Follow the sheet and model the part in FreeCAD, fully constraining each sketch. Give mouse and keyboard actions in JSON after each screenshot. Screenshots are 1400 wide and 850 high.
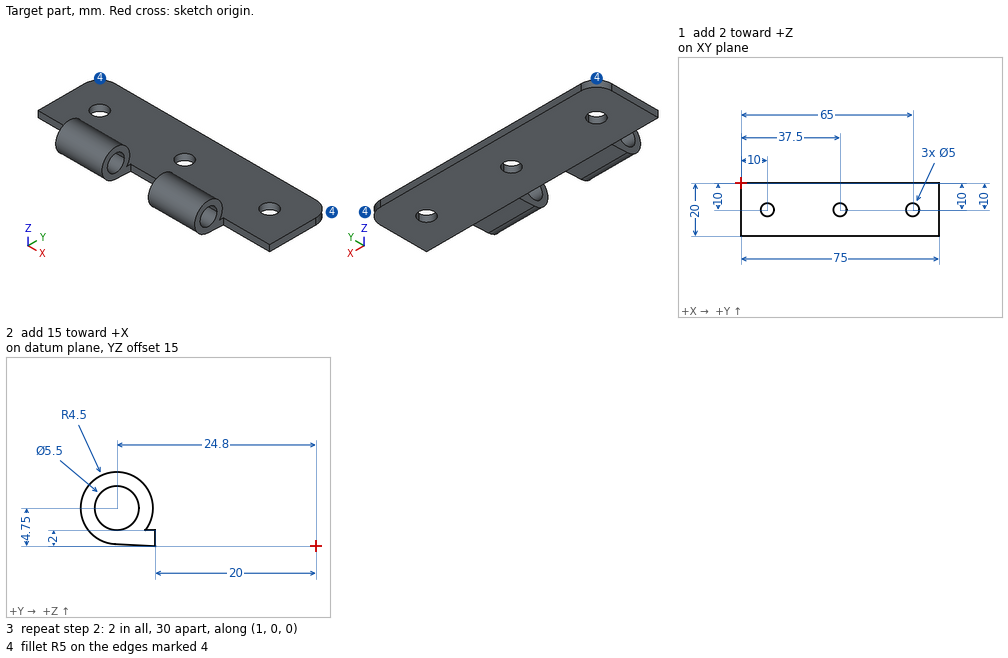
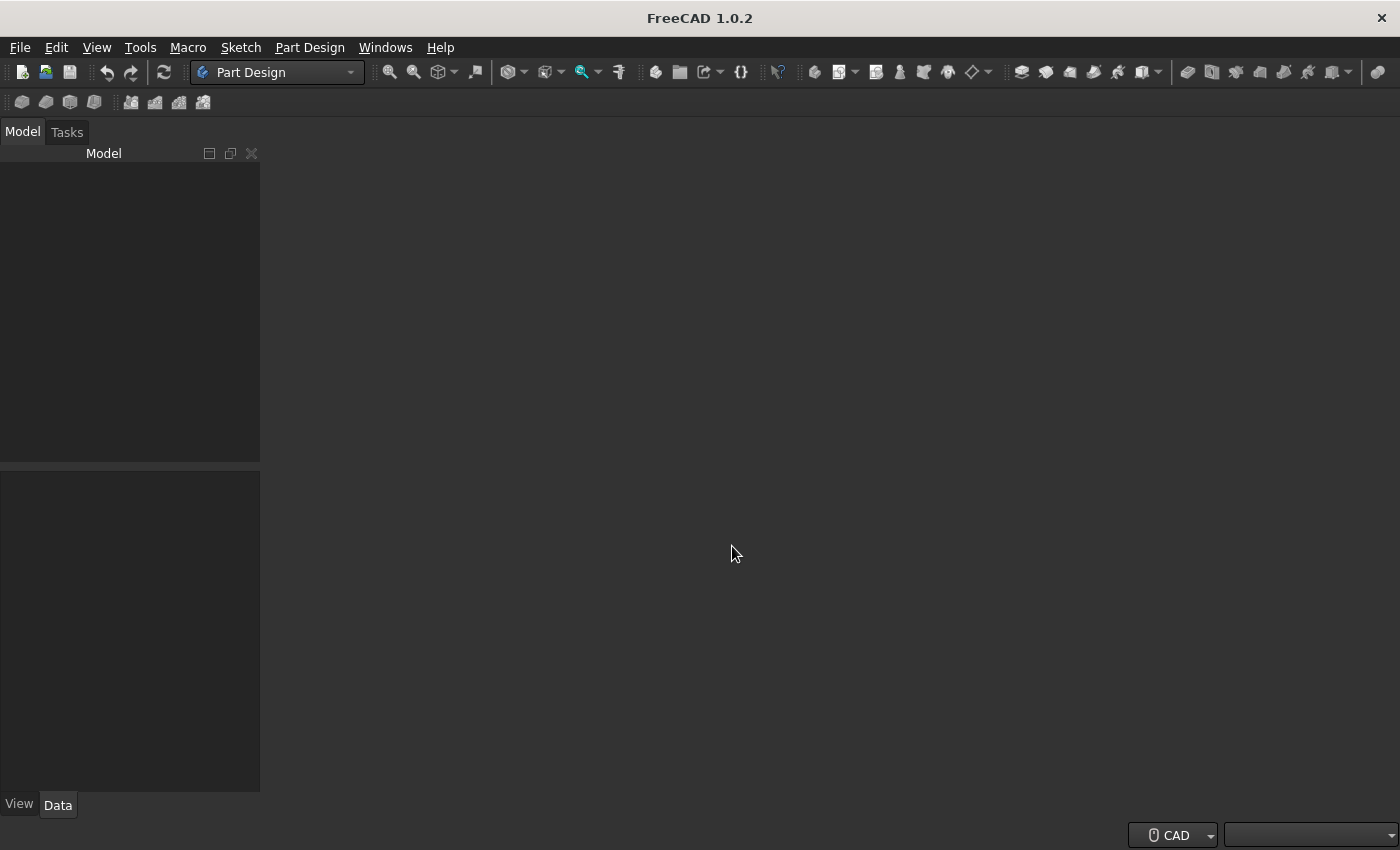
{"action": "left_click", "coordinate": [22, 72]}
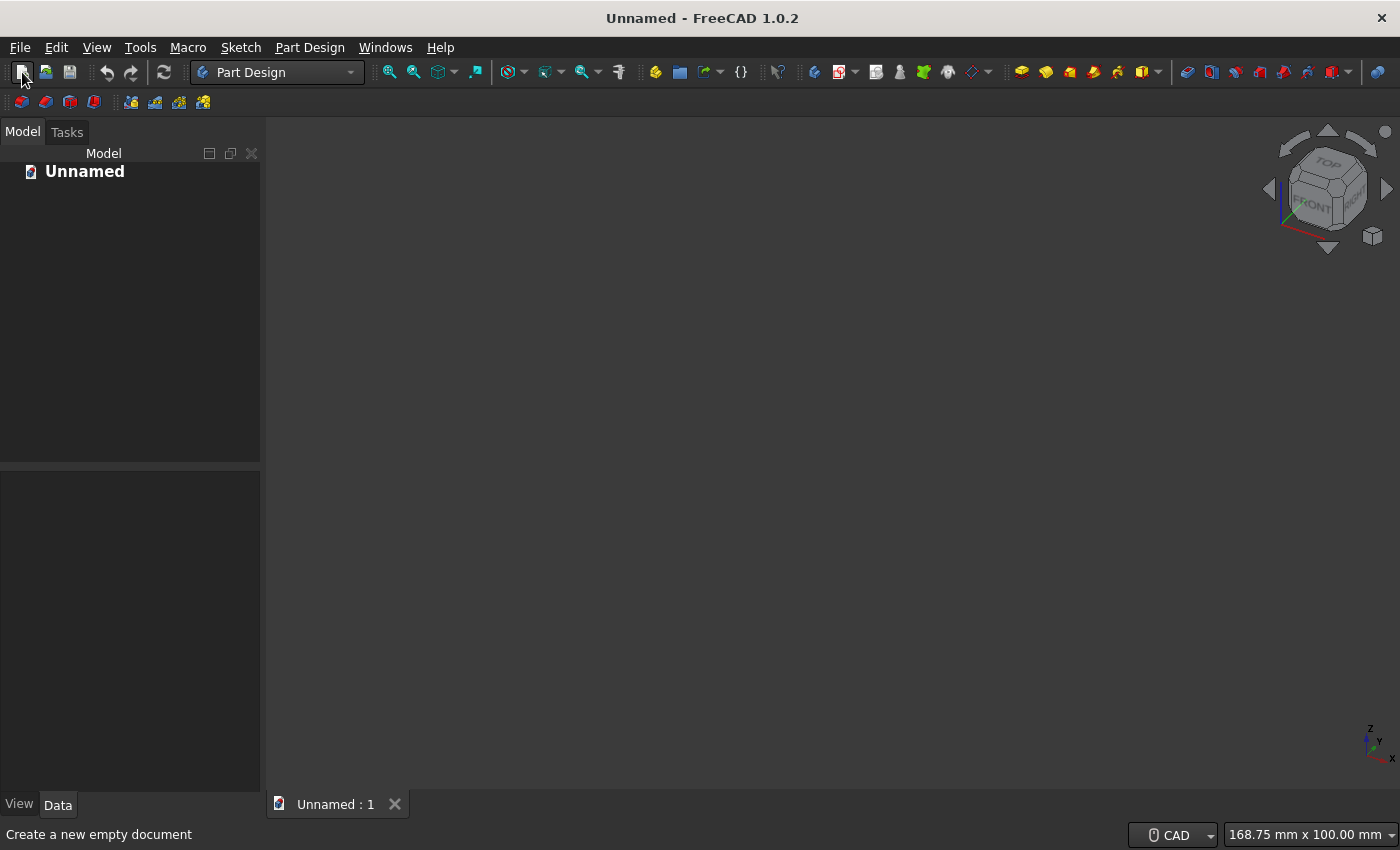
{"action": "left_click", "coordinate": [840, 72]}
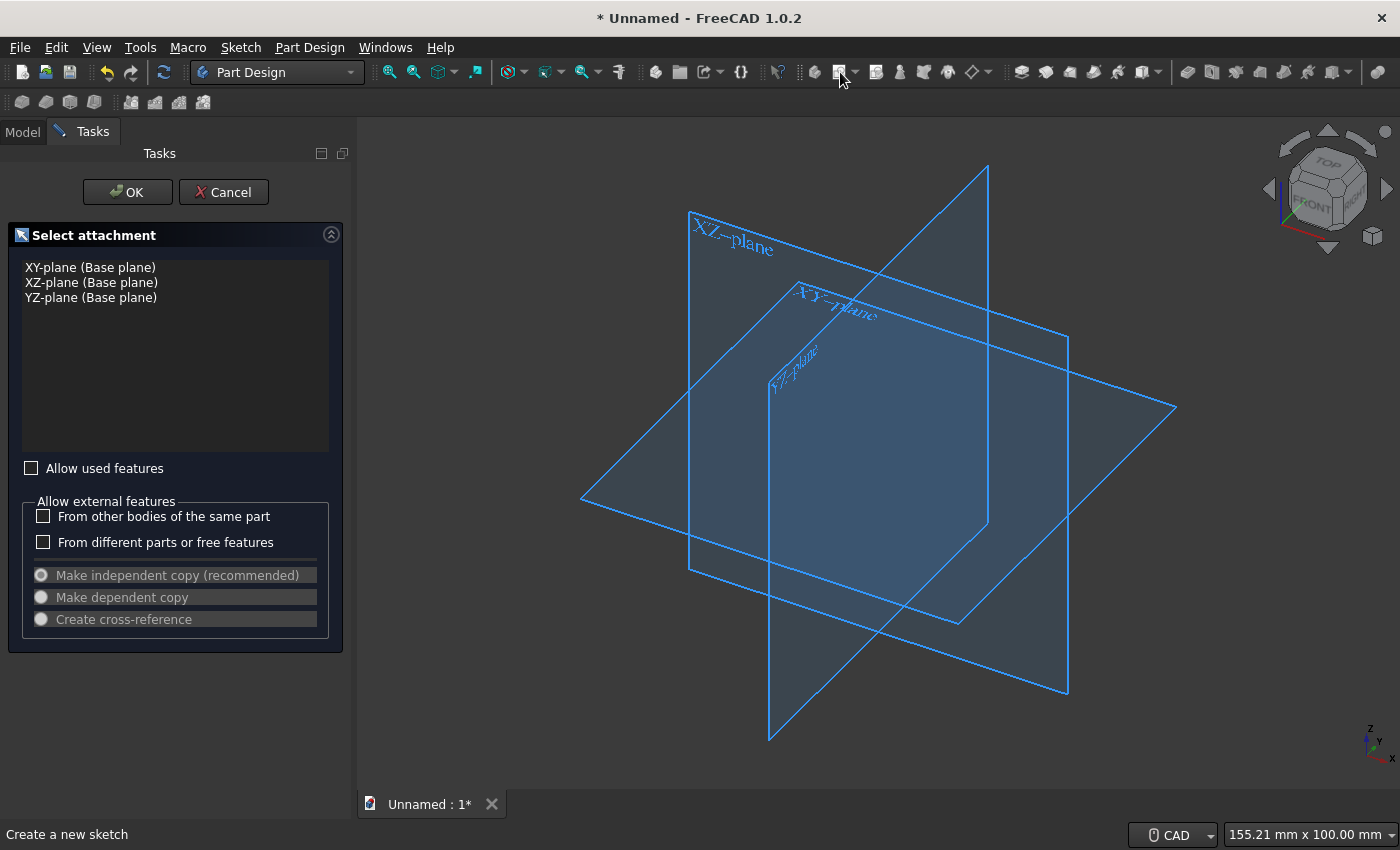
{"action": "left_click", "coordinate": [82, 268]}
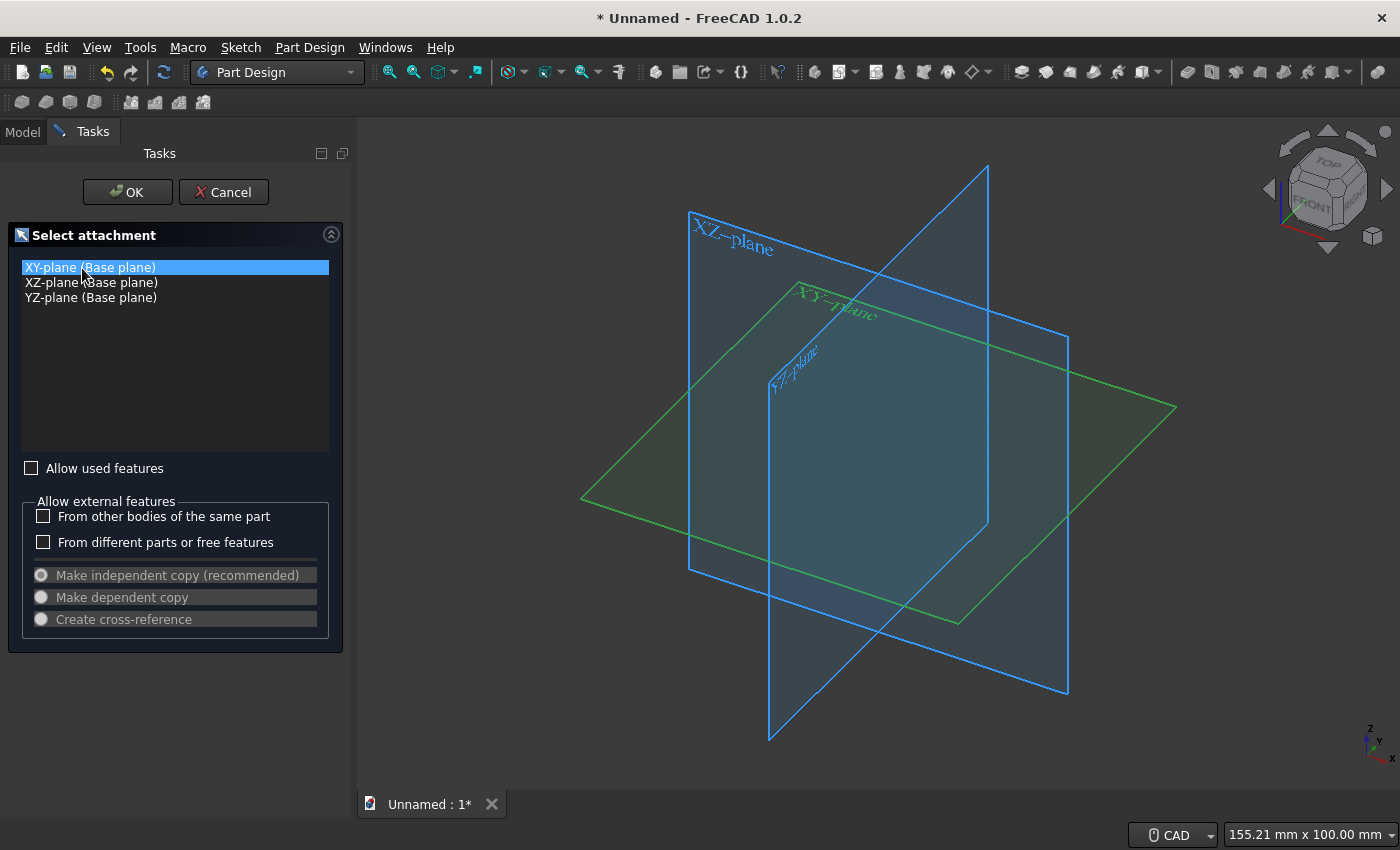
{"action": "left_click", "coordinate": [128, 192]}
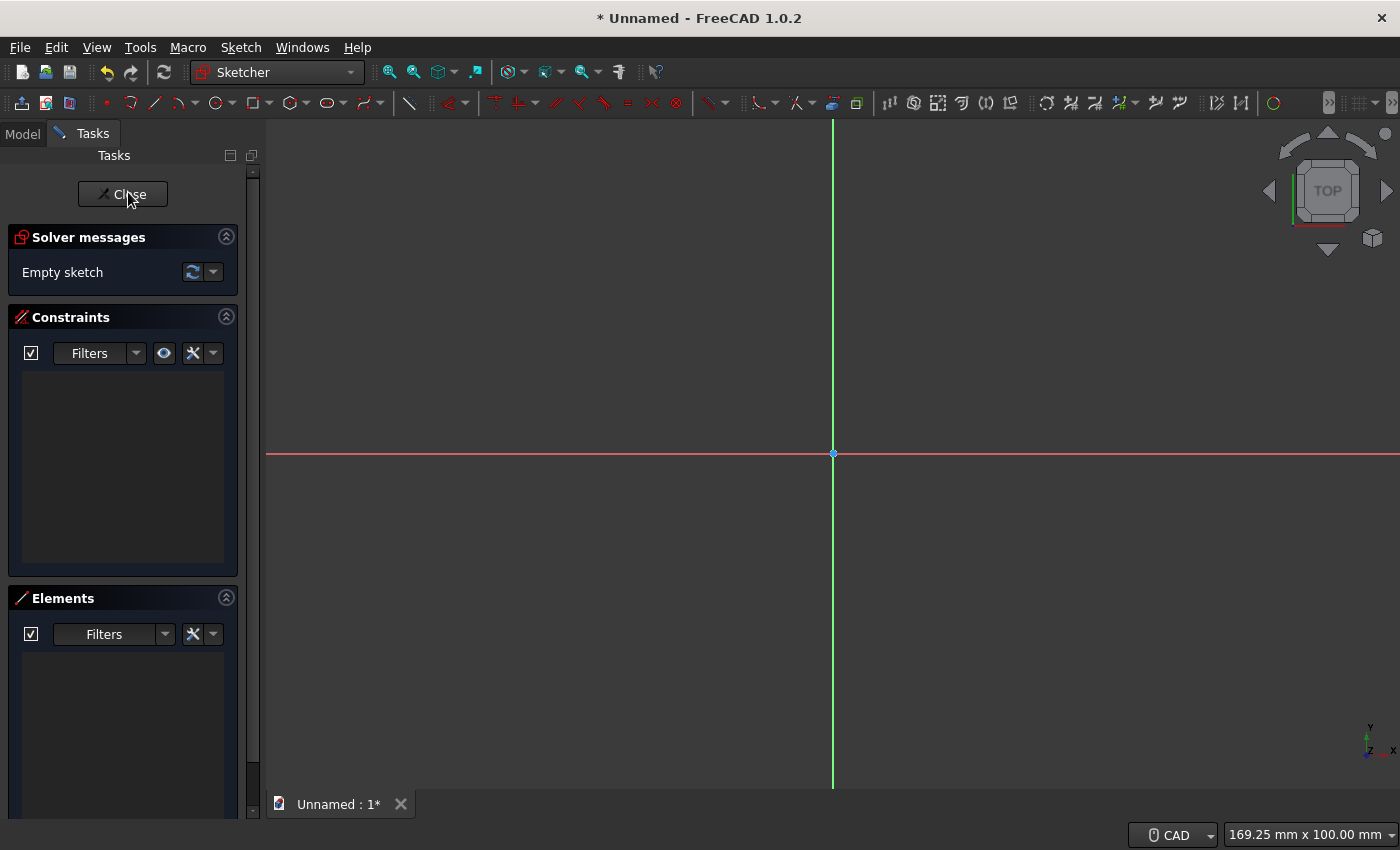
{"action": "scroll", "coordinate": [294, 151], "scroll_direction": "down", "scroll_amount": 1}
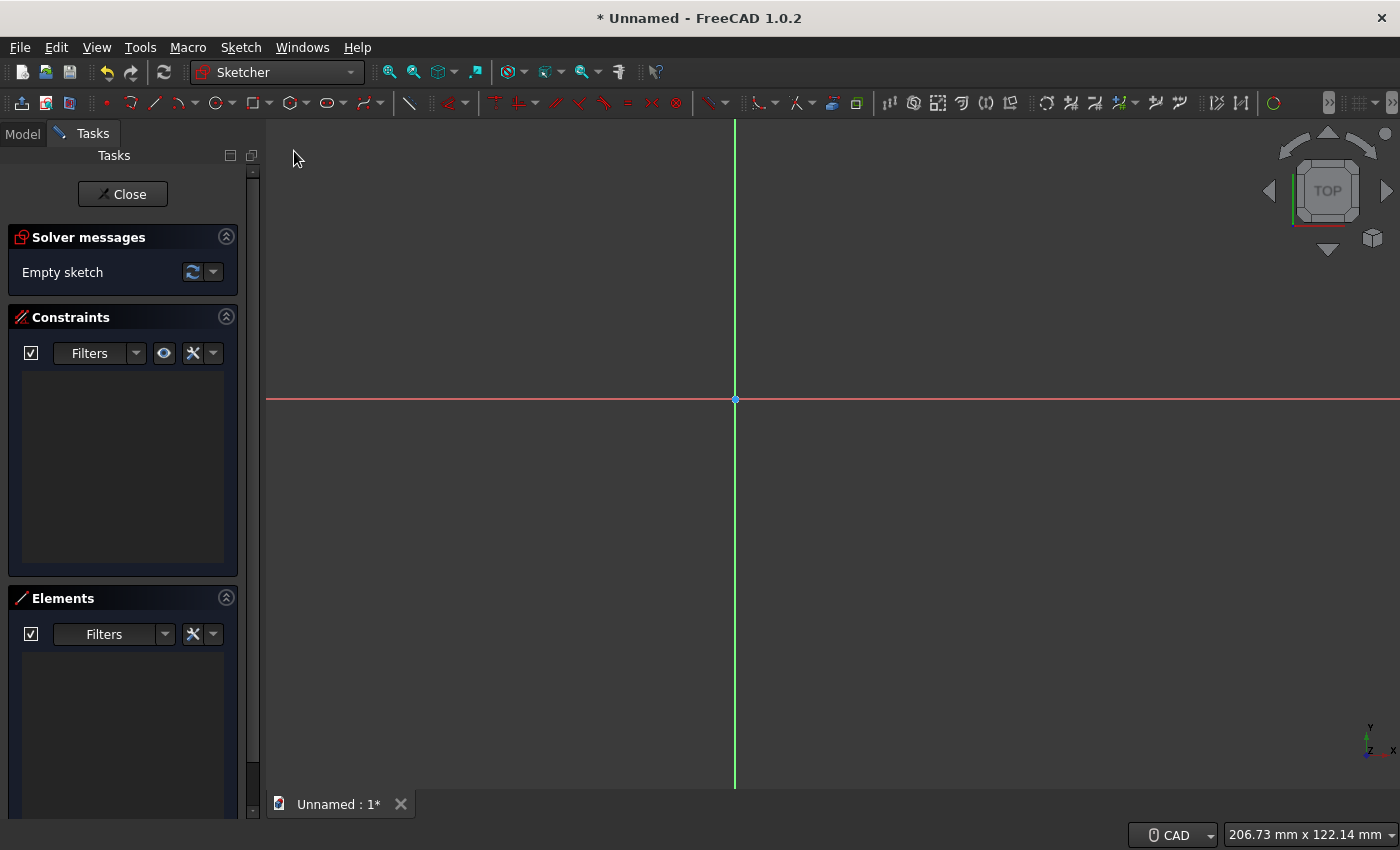
{"action": "scroll", "coordinate": [1235, 454], "scroll_direction": "up", "scroll_amount": 2}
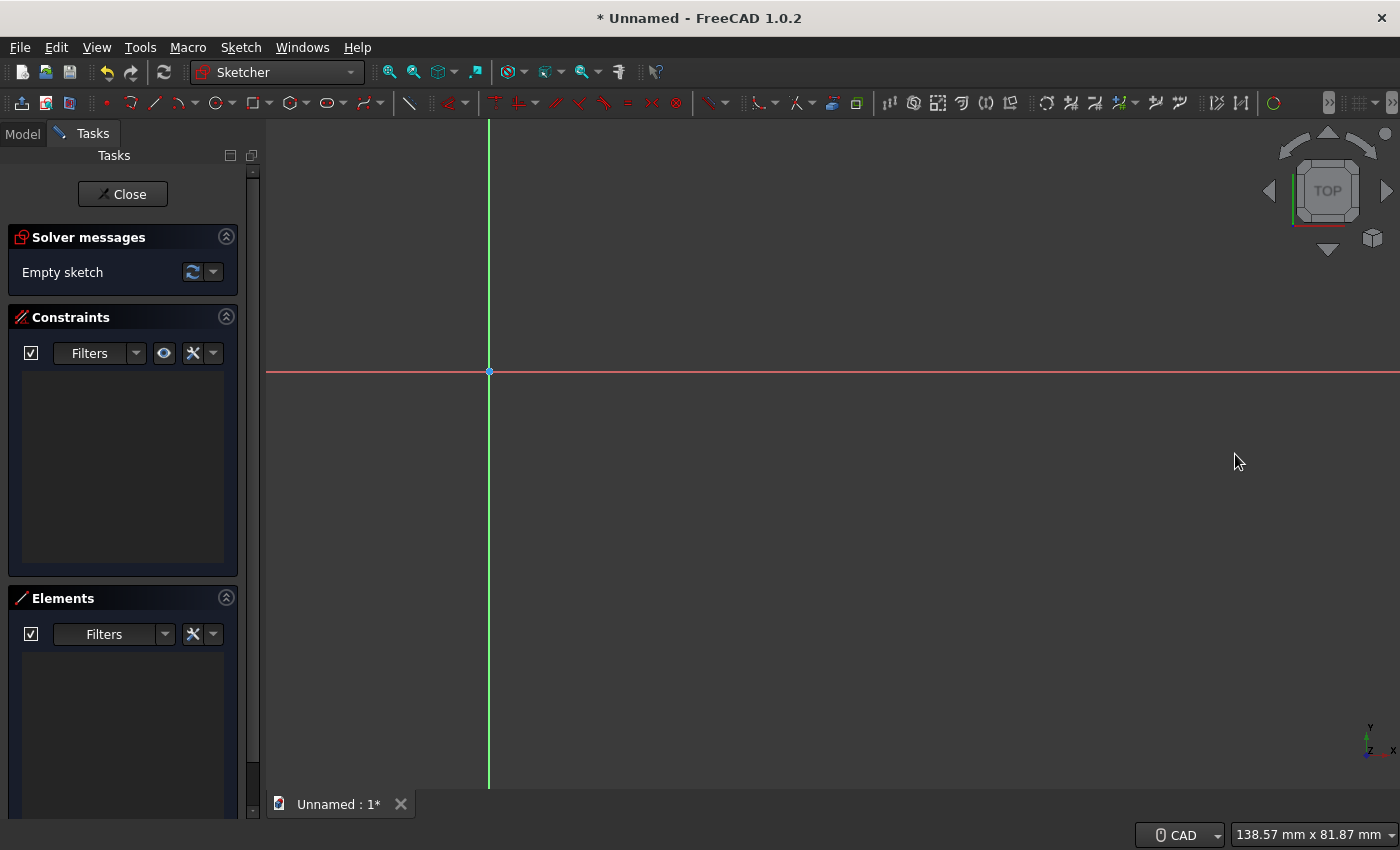
{"action": "key", "text": "g r"}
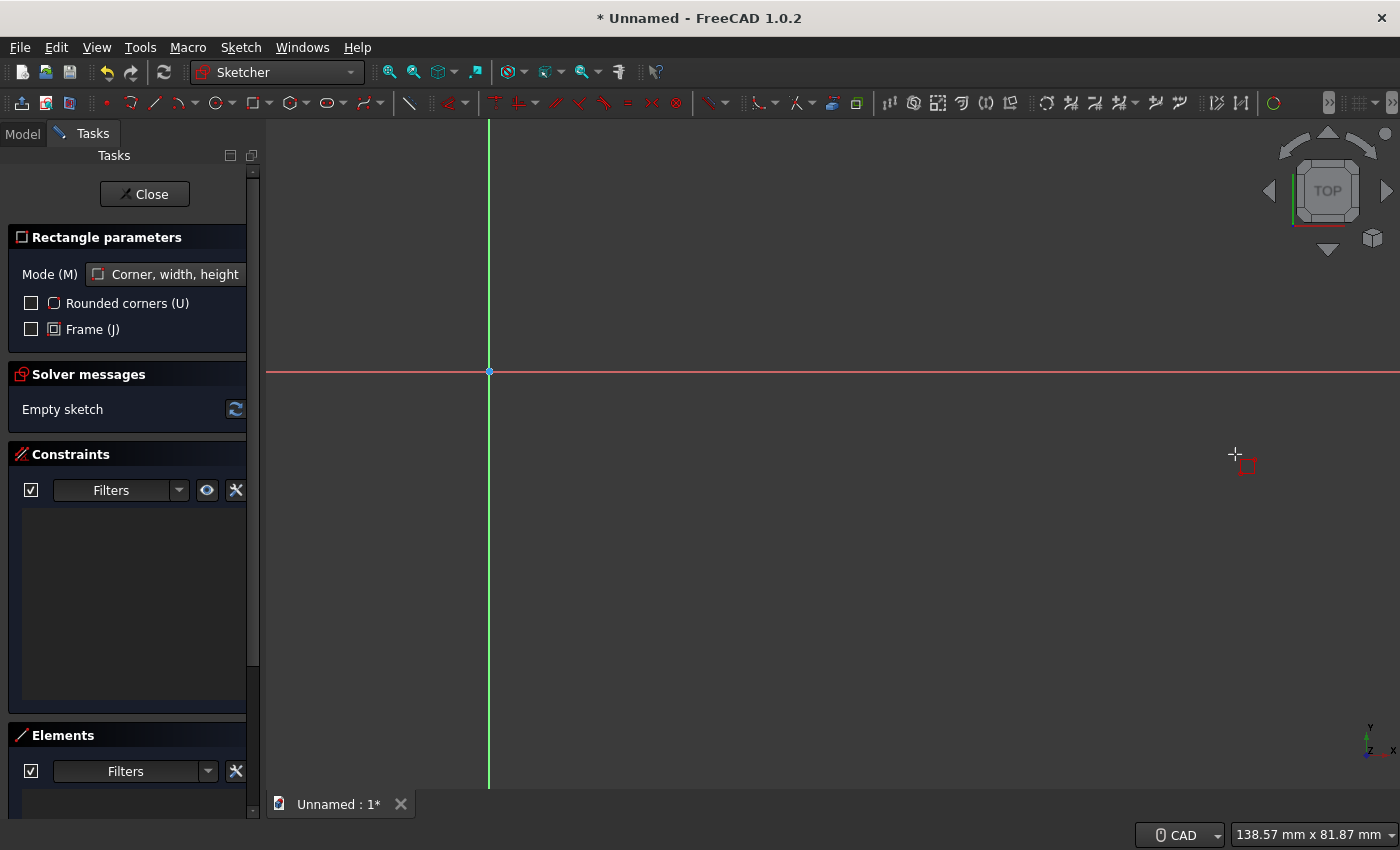
{"action": "left_click", "coordinate": [489, 372]}
{"action": "left_click", "coordinate": [1103, 535]}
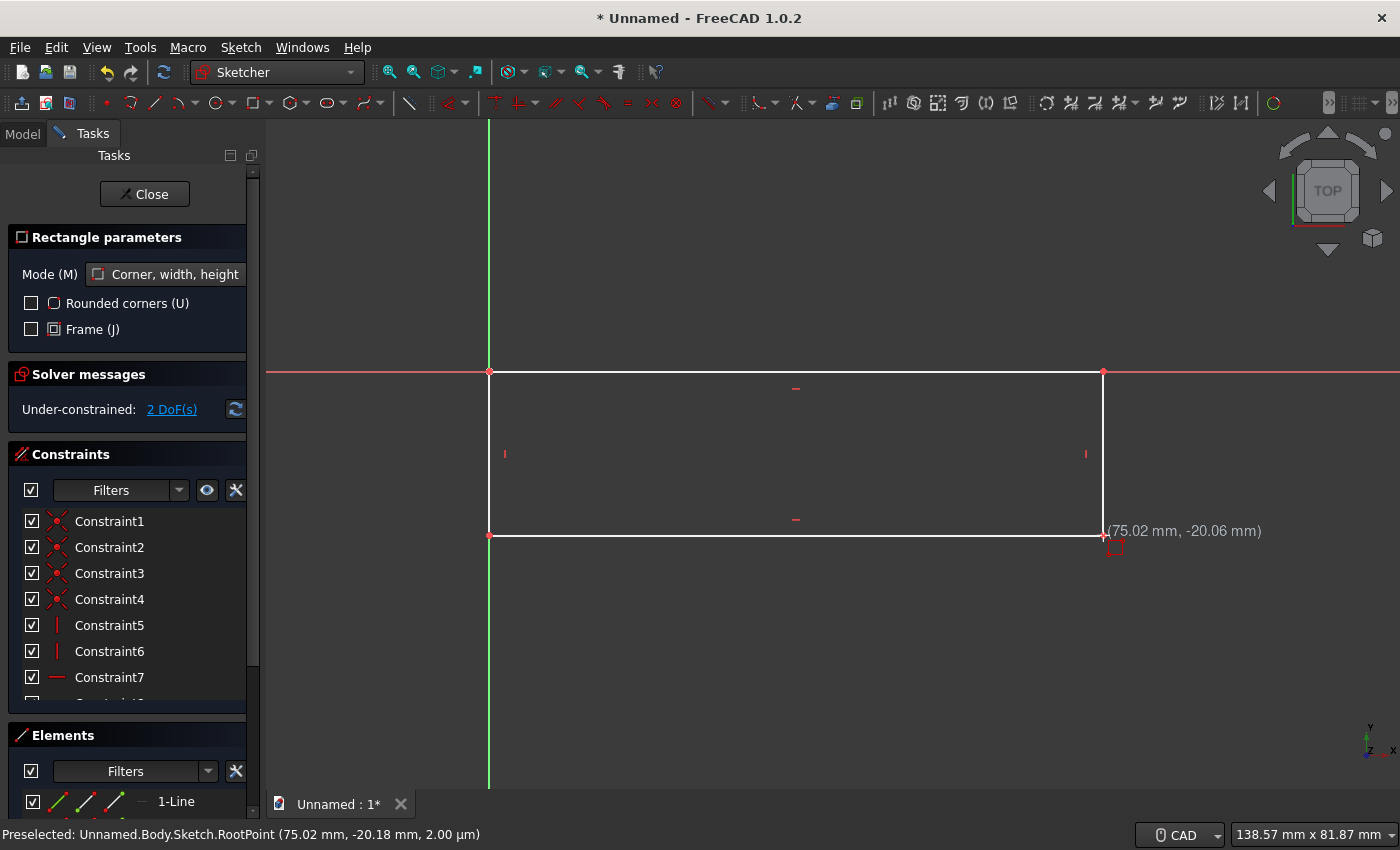
{"action": "key", "text": "g c"}